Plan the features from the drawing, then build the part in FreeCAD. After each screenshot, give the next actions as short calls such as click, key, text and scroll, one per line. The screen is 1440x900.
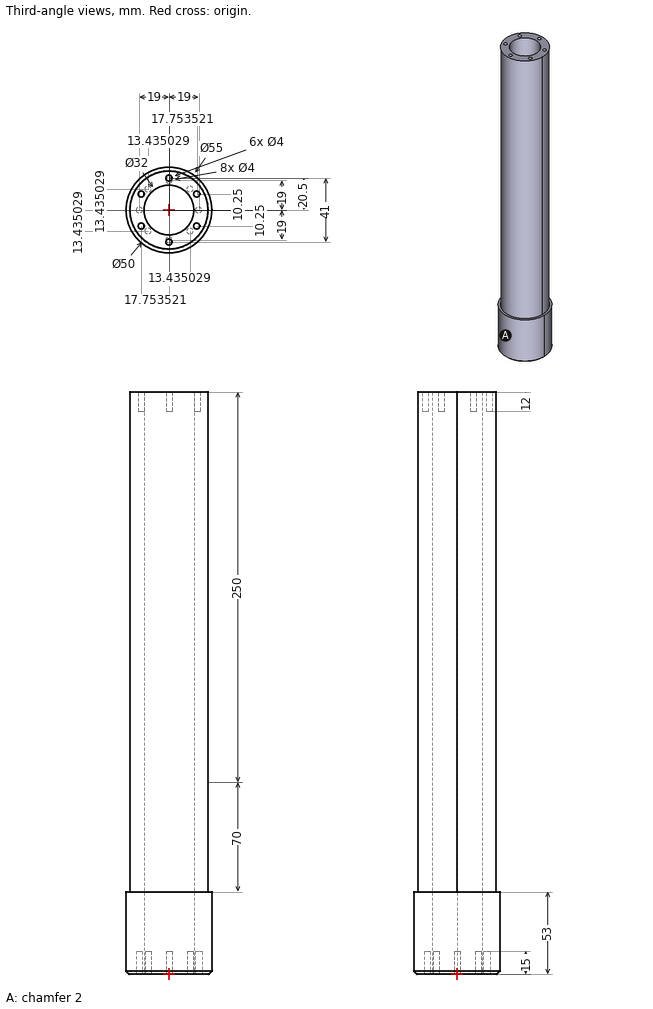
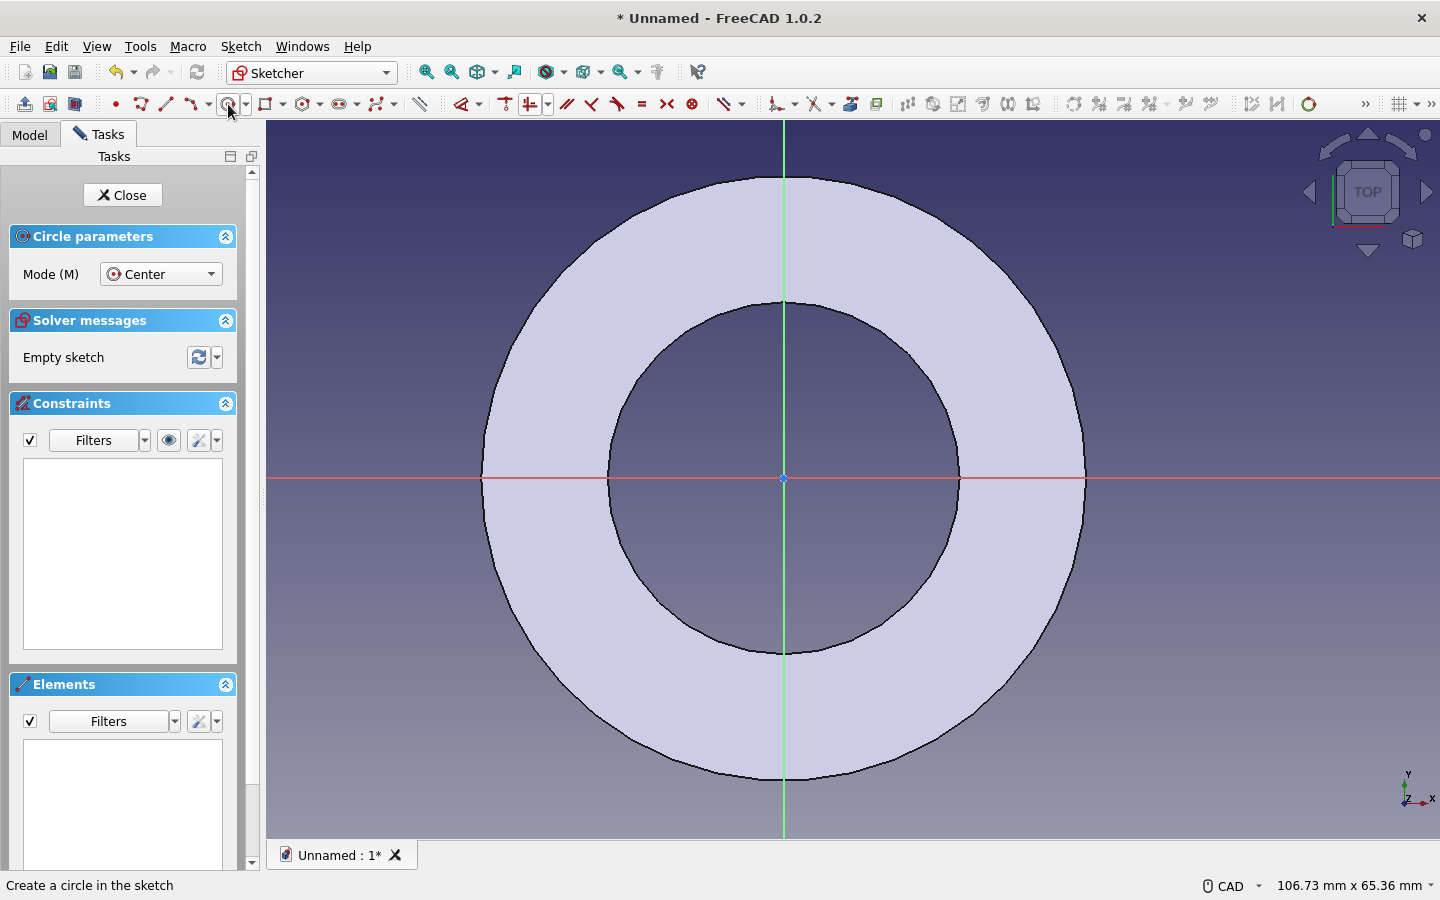
click(784, 269)
move(799, 254)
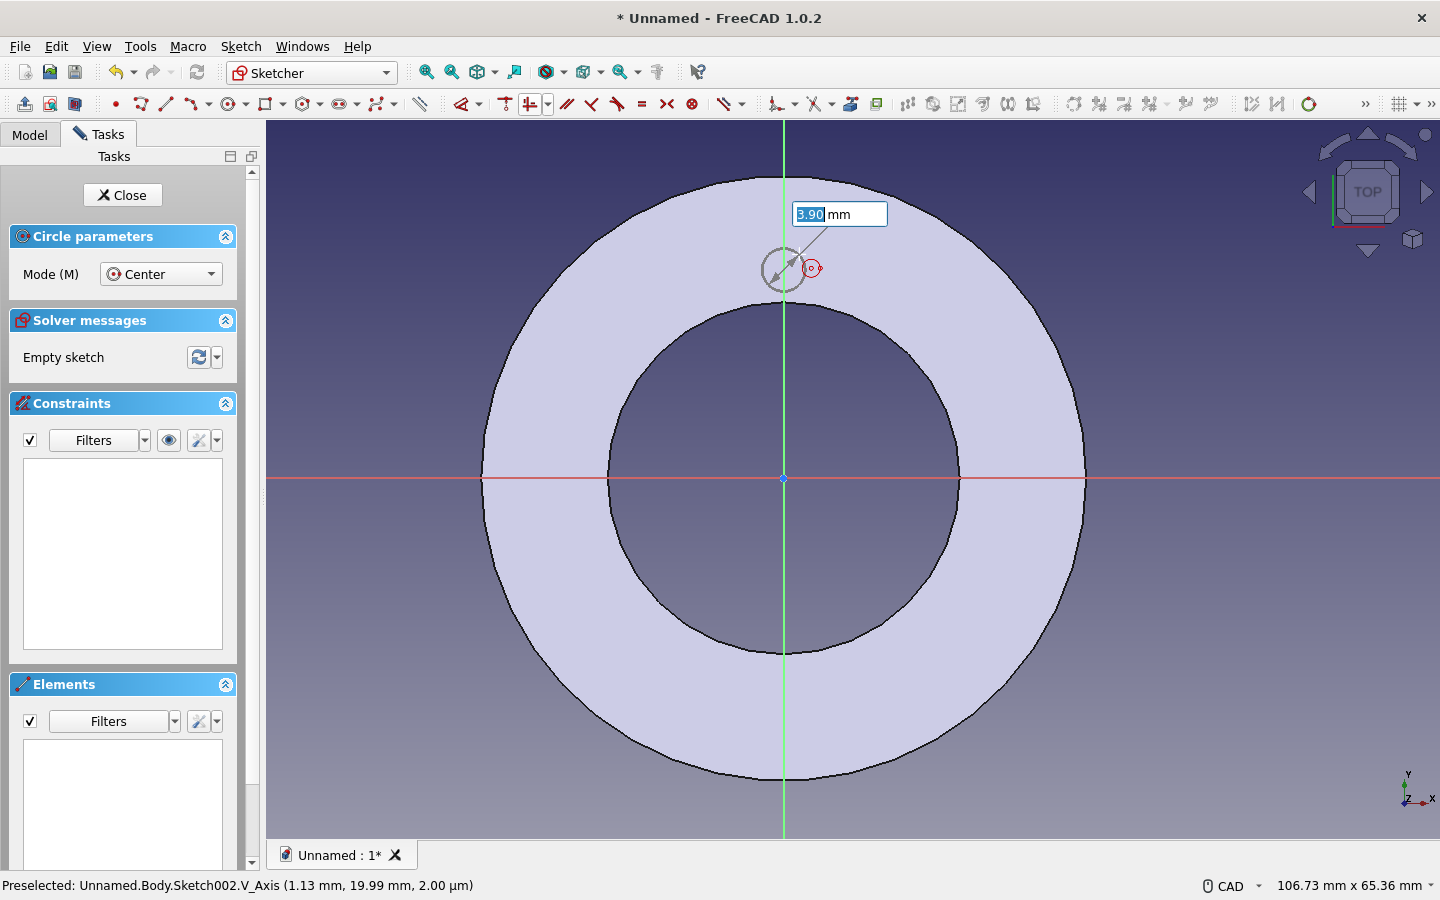
text(4)
key(Return)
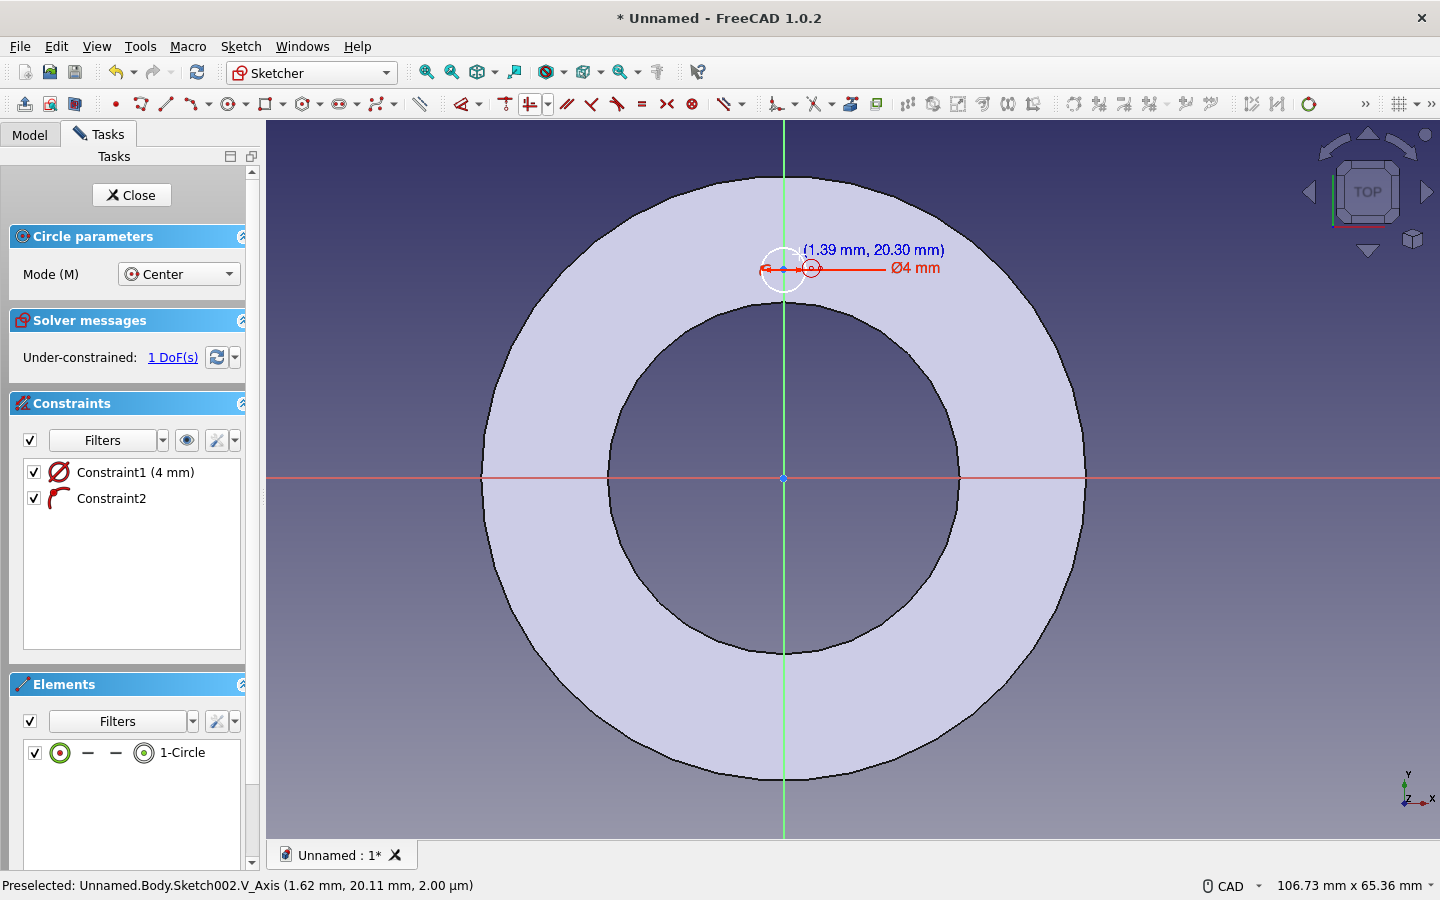
click(636, 330)
move(651, 315)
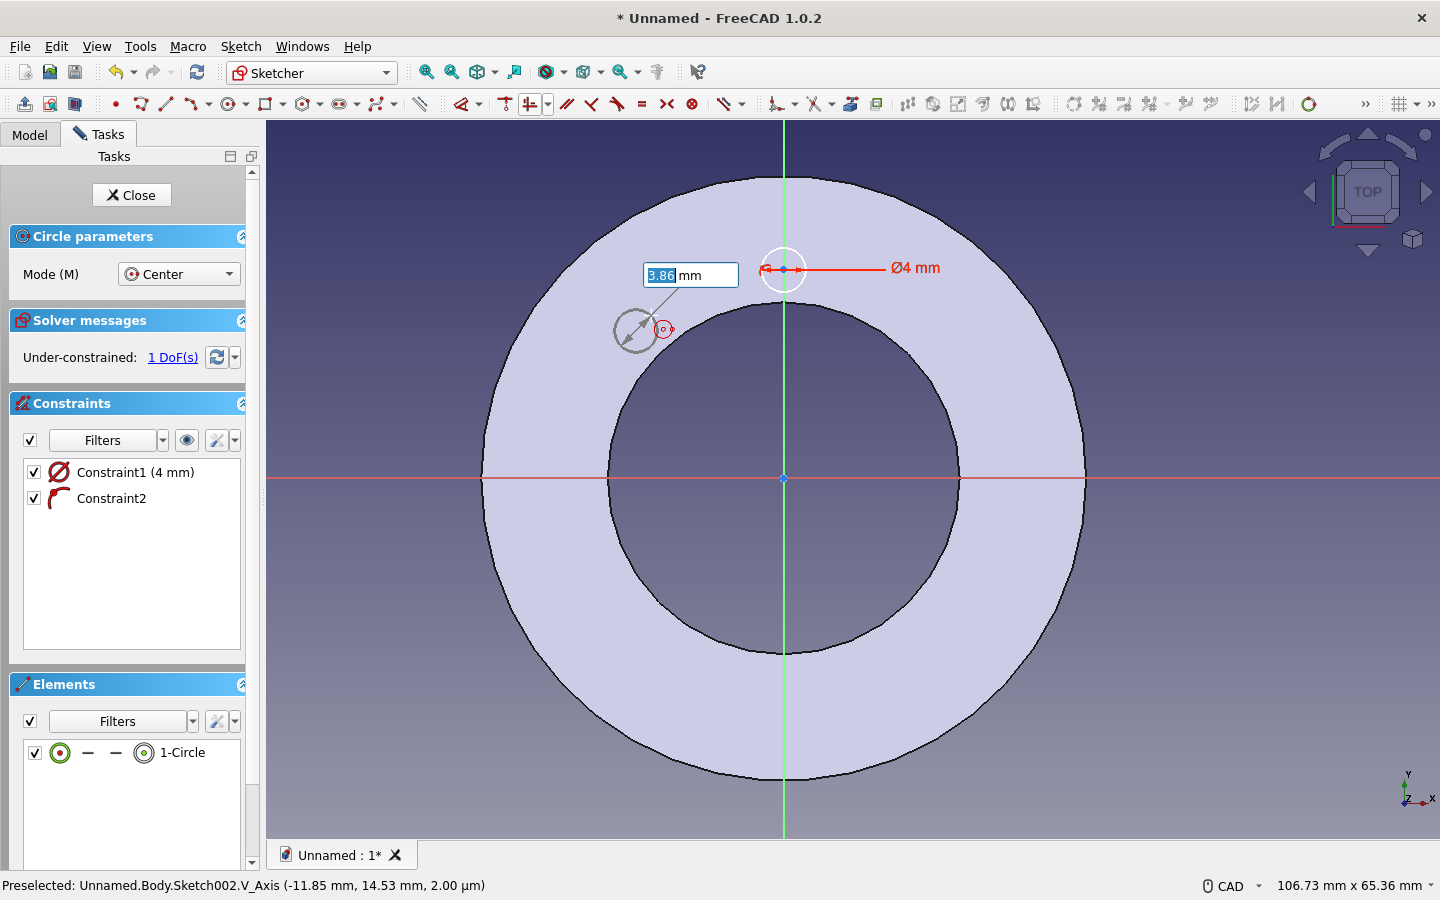
text(4)
key(Return)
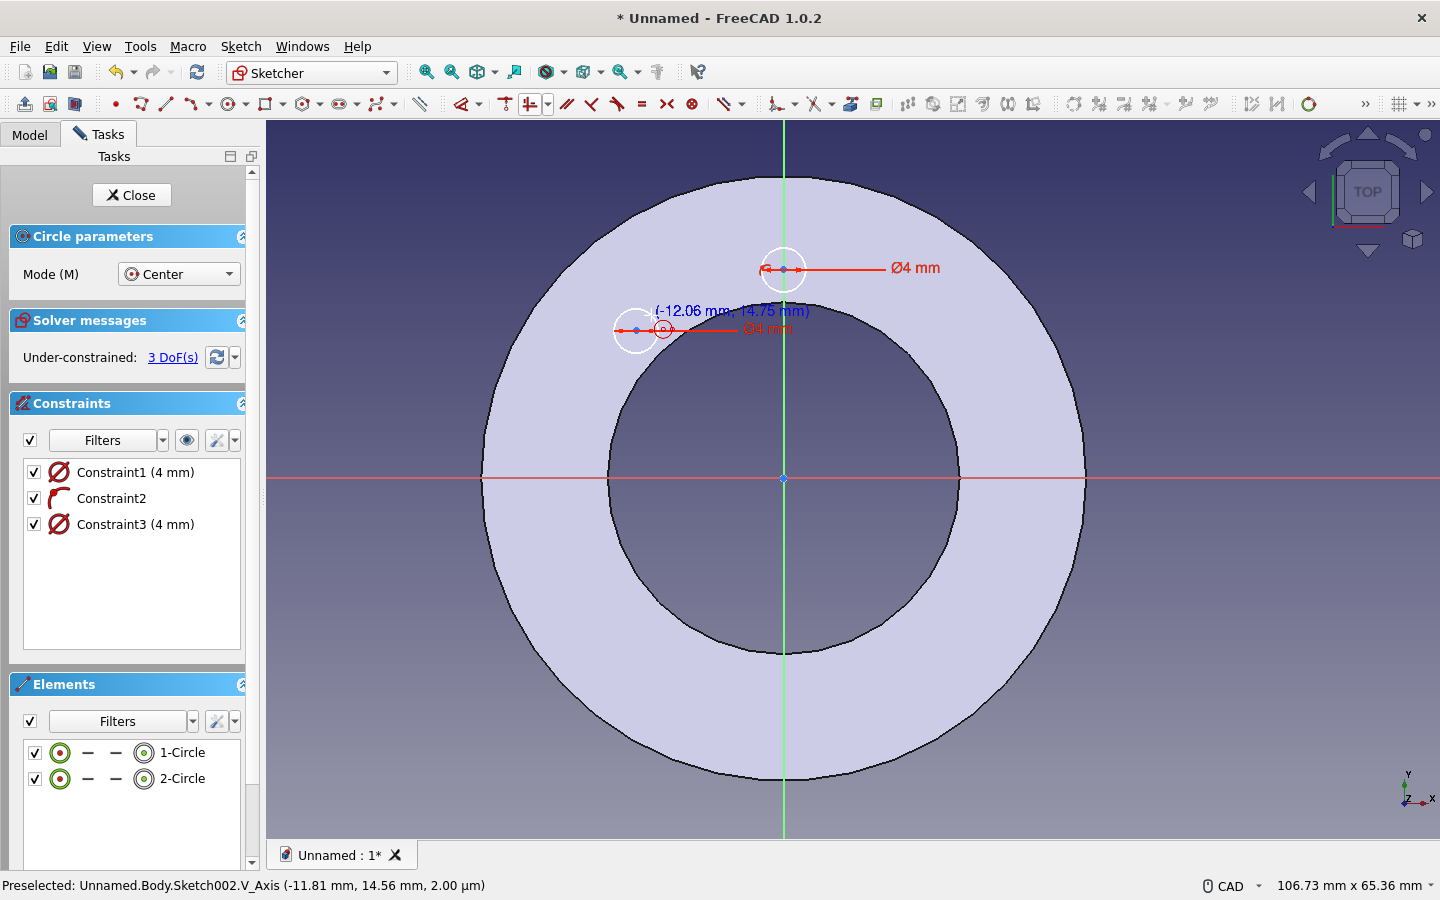
click(575, 478)
move(590, 463)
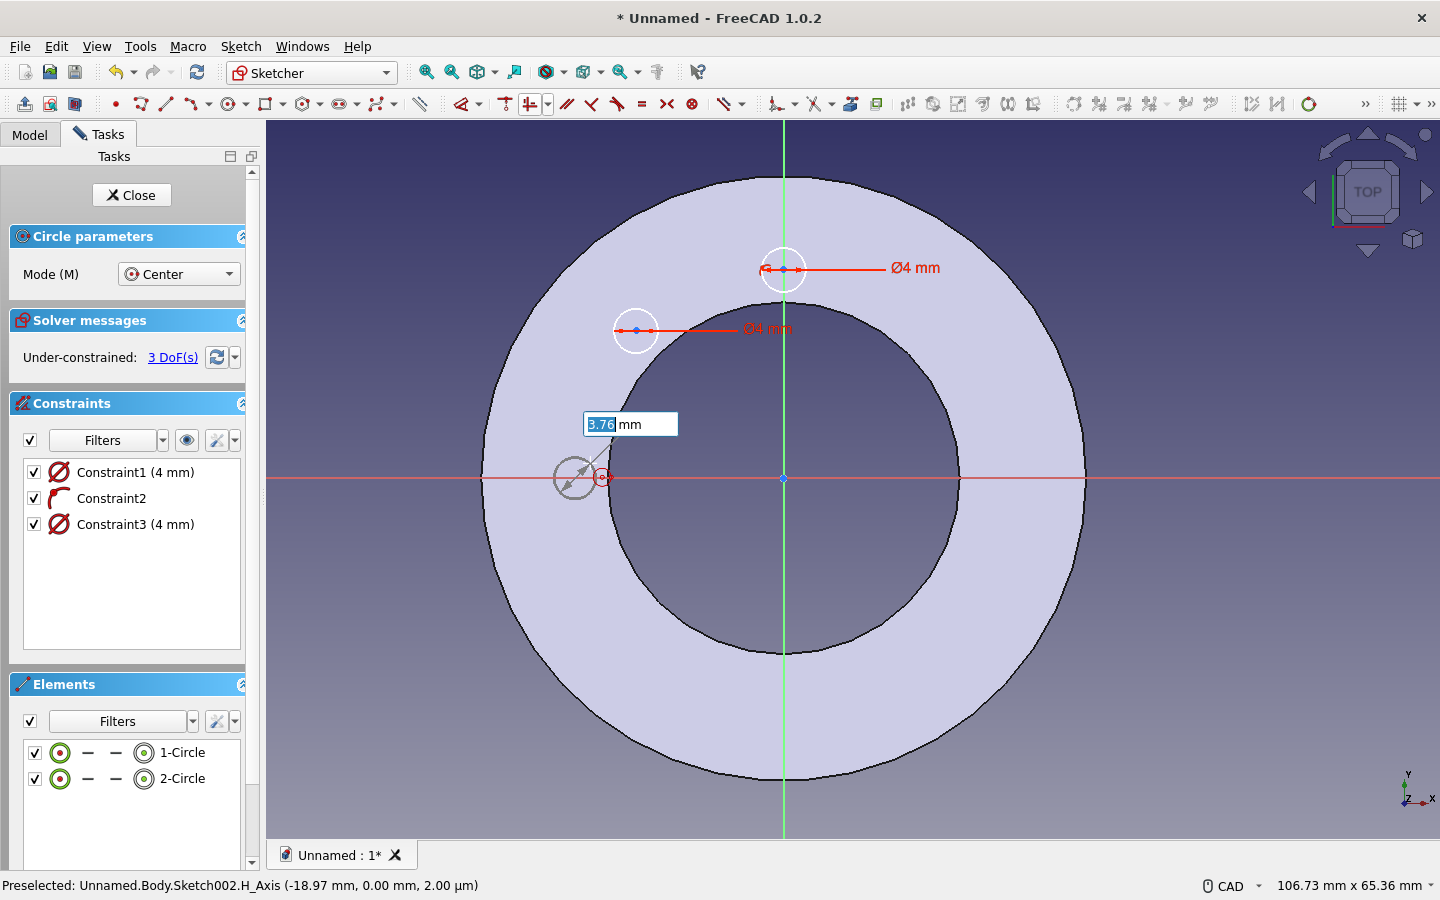
text(4)
key(Return)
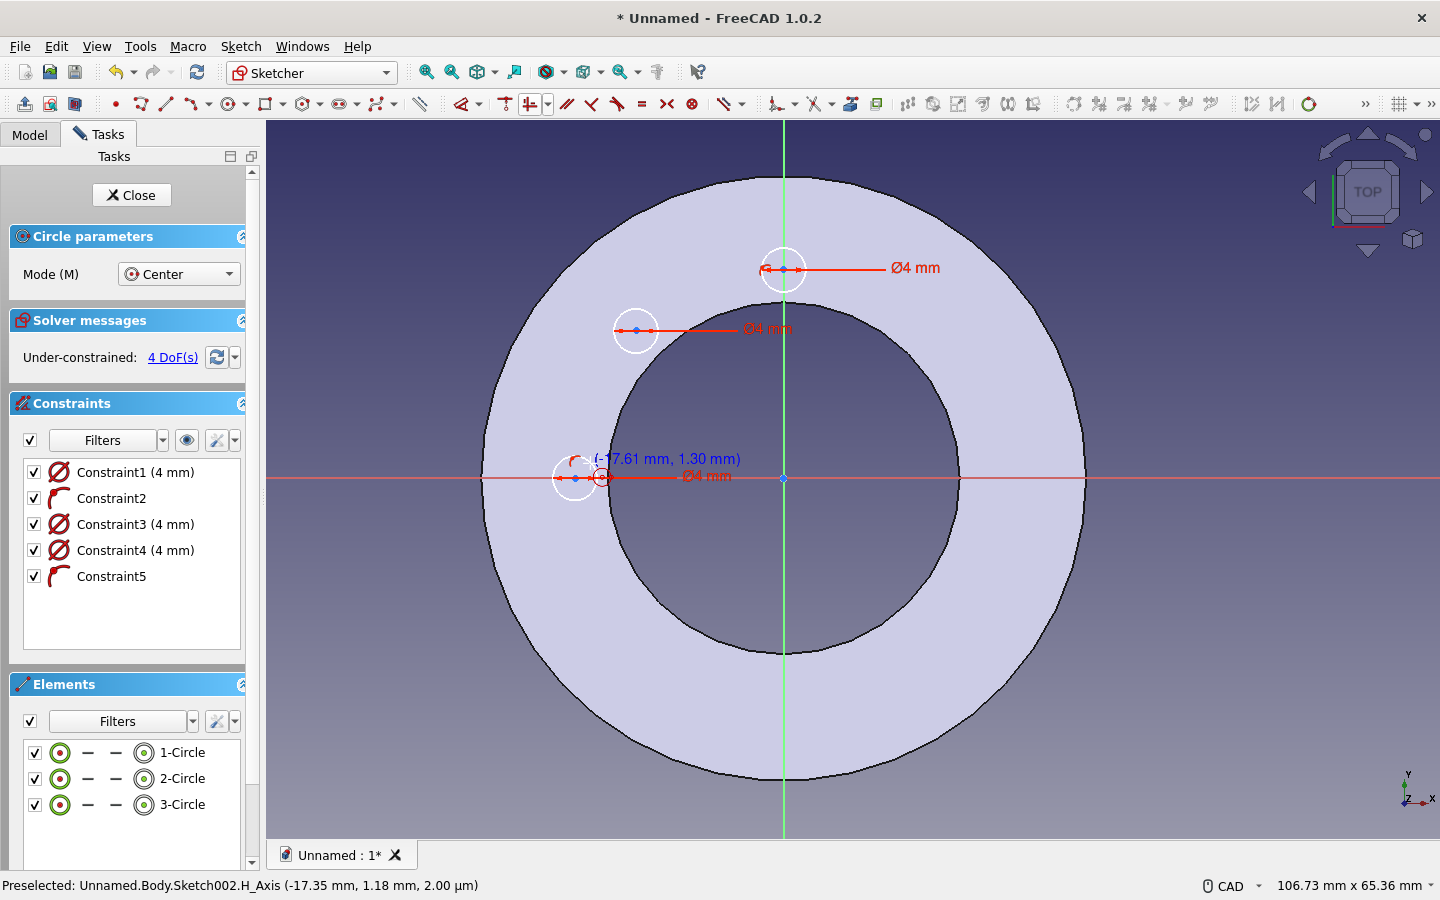
click(636, 626)
move(651, 610)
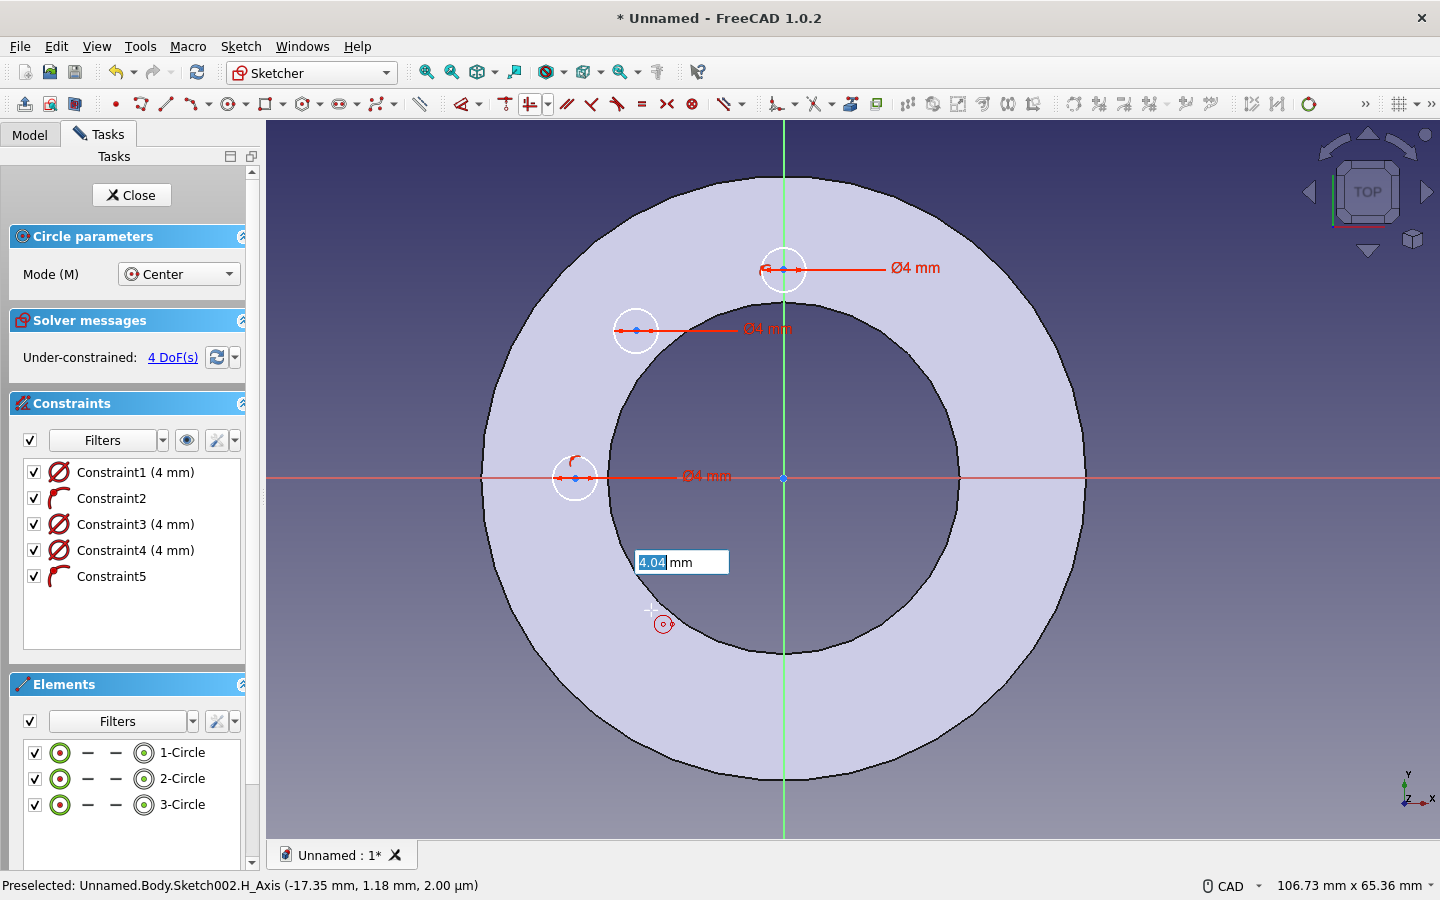
text(4)
key(Return)